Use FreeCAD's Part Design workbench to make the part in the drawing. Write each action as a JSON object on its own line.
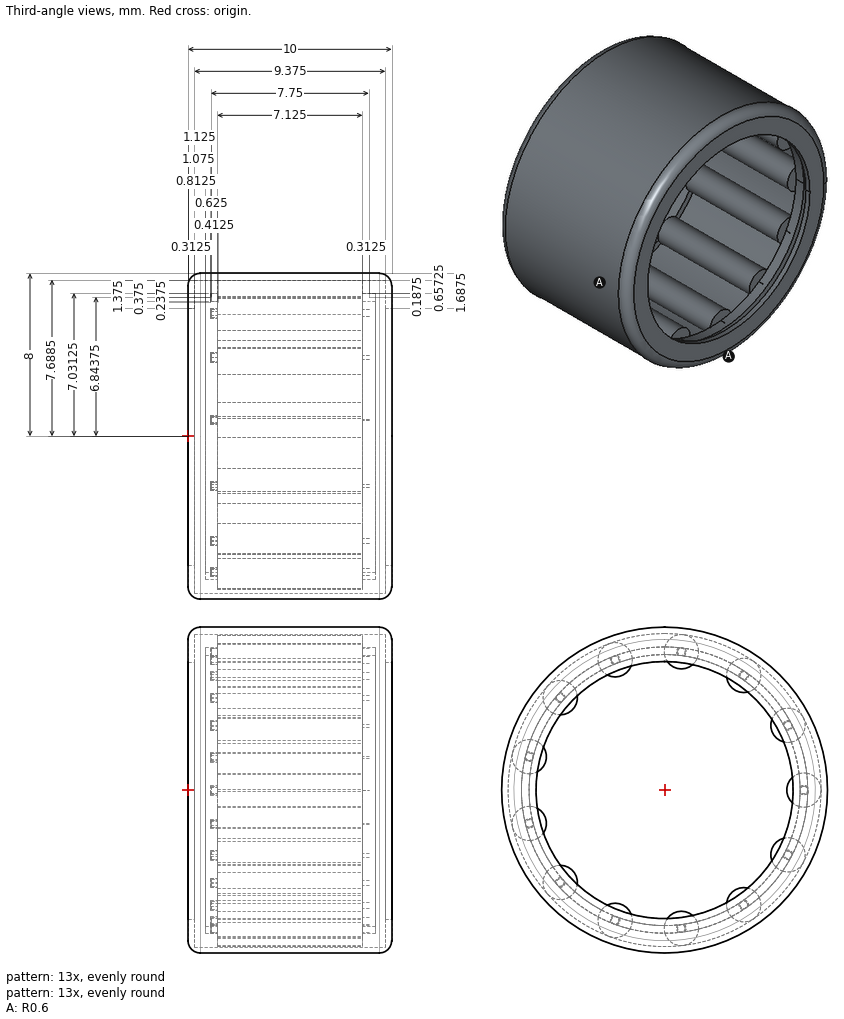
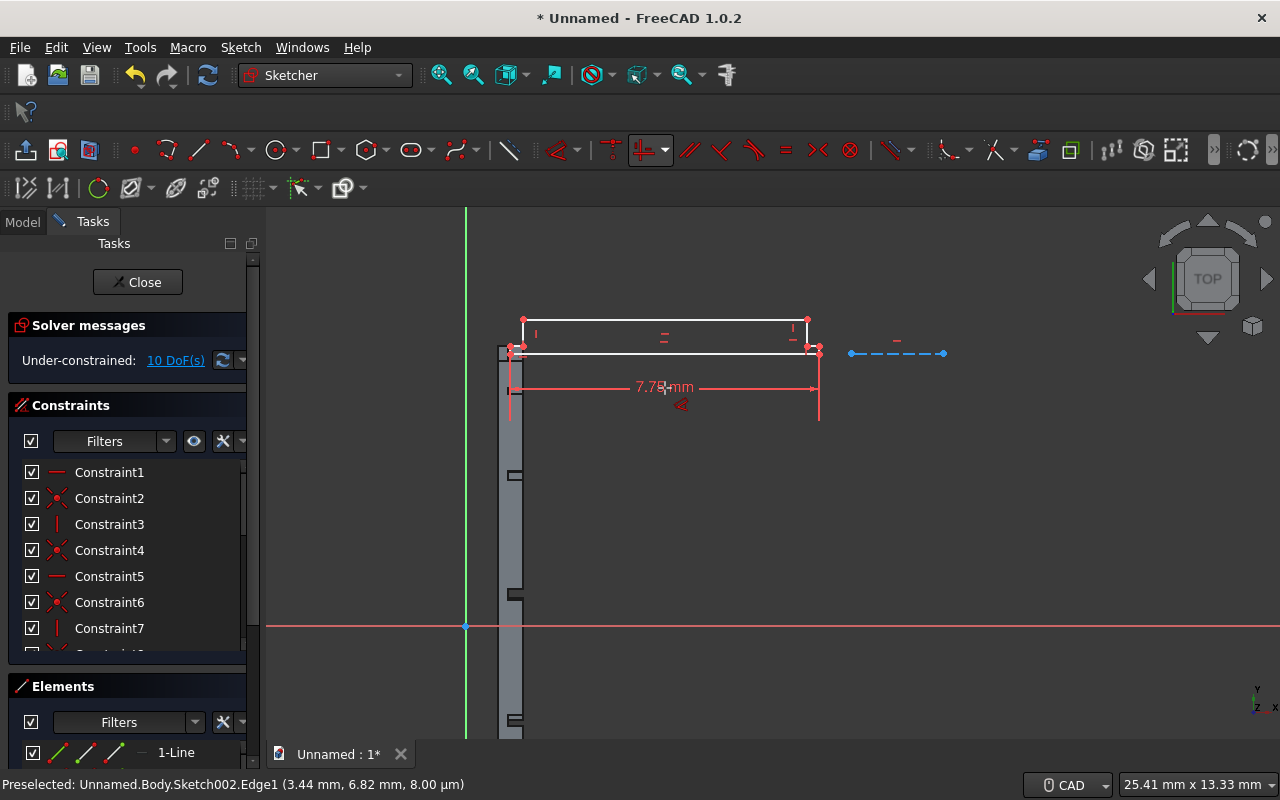
{"action": "left_click", "coordinate": [722, 320]}
{"action": "left_click", "coordinate": [665, 286]}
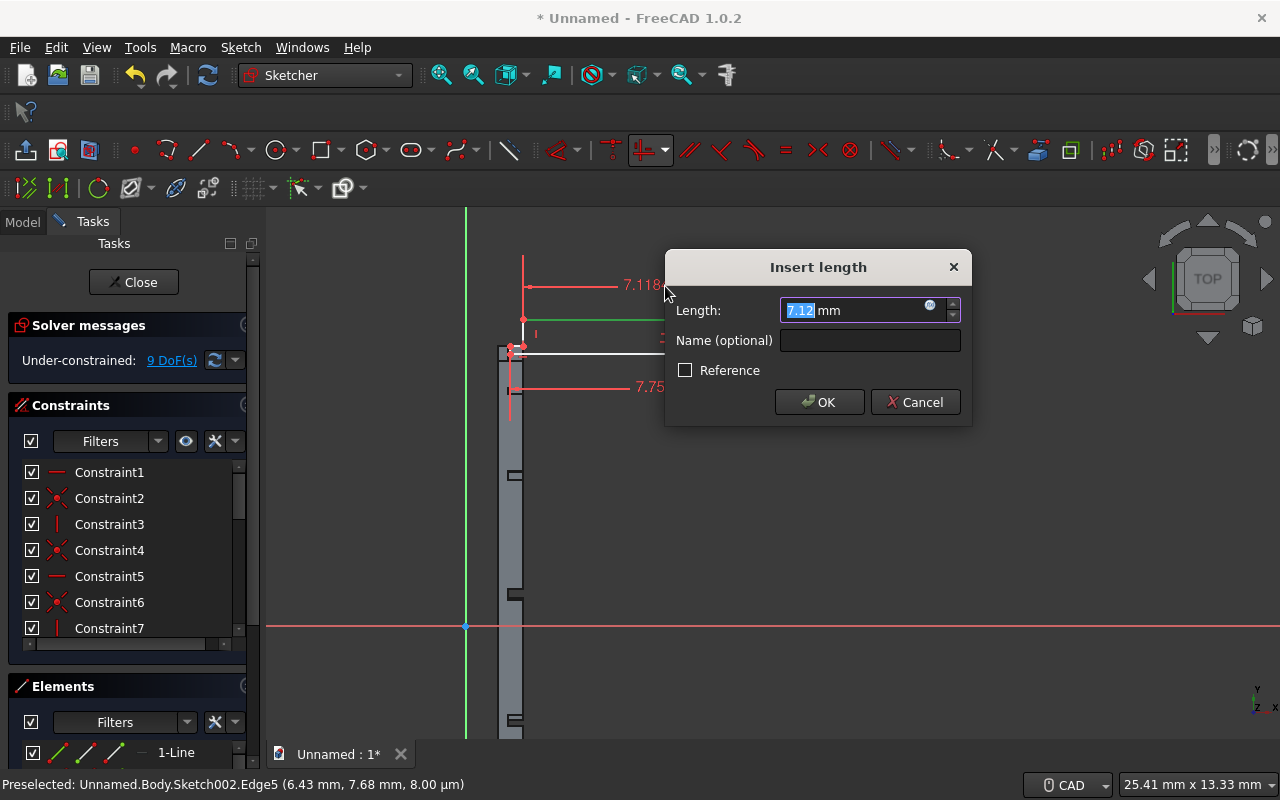
{"action": "type", "text": "7.125"}
{"action": "key", "text": "Return"}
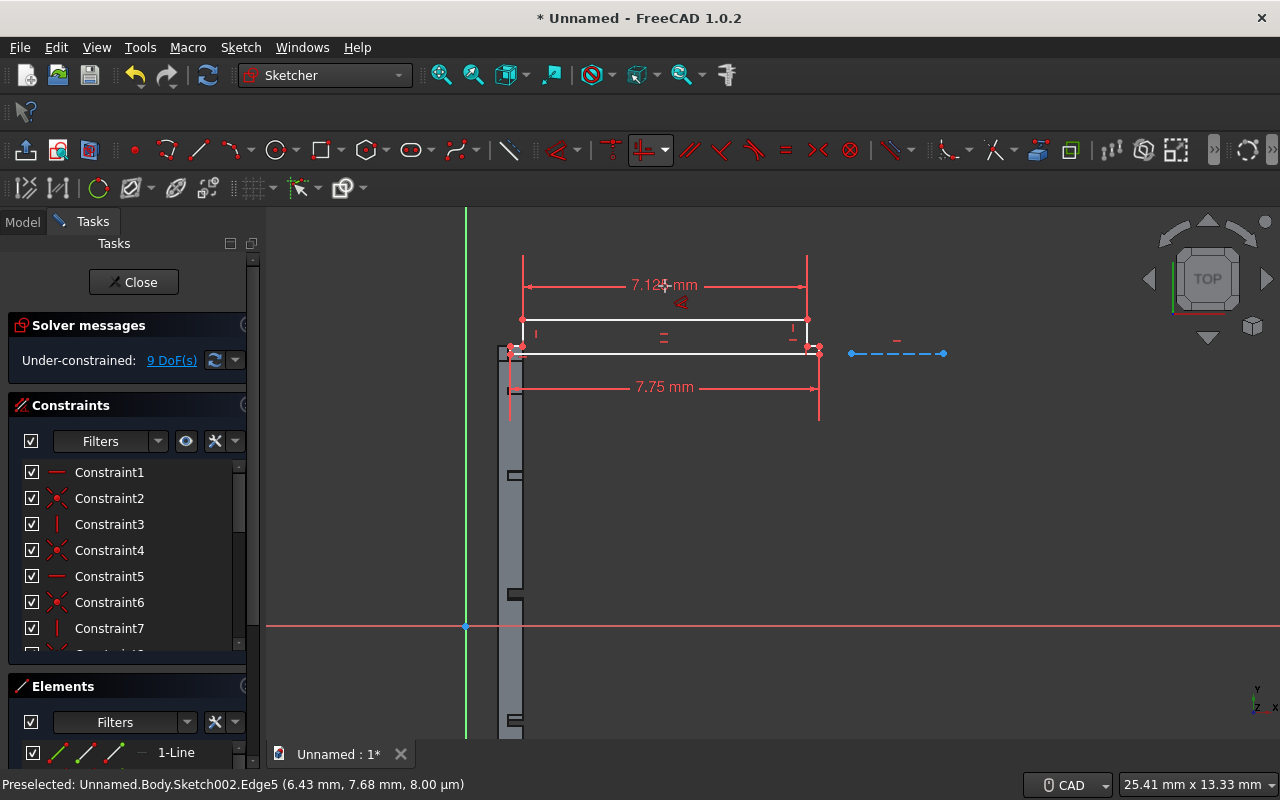
{"action": "scroll", "coordinate": [819, 350], "scroll_direction": "up", "scroll_amount": 9}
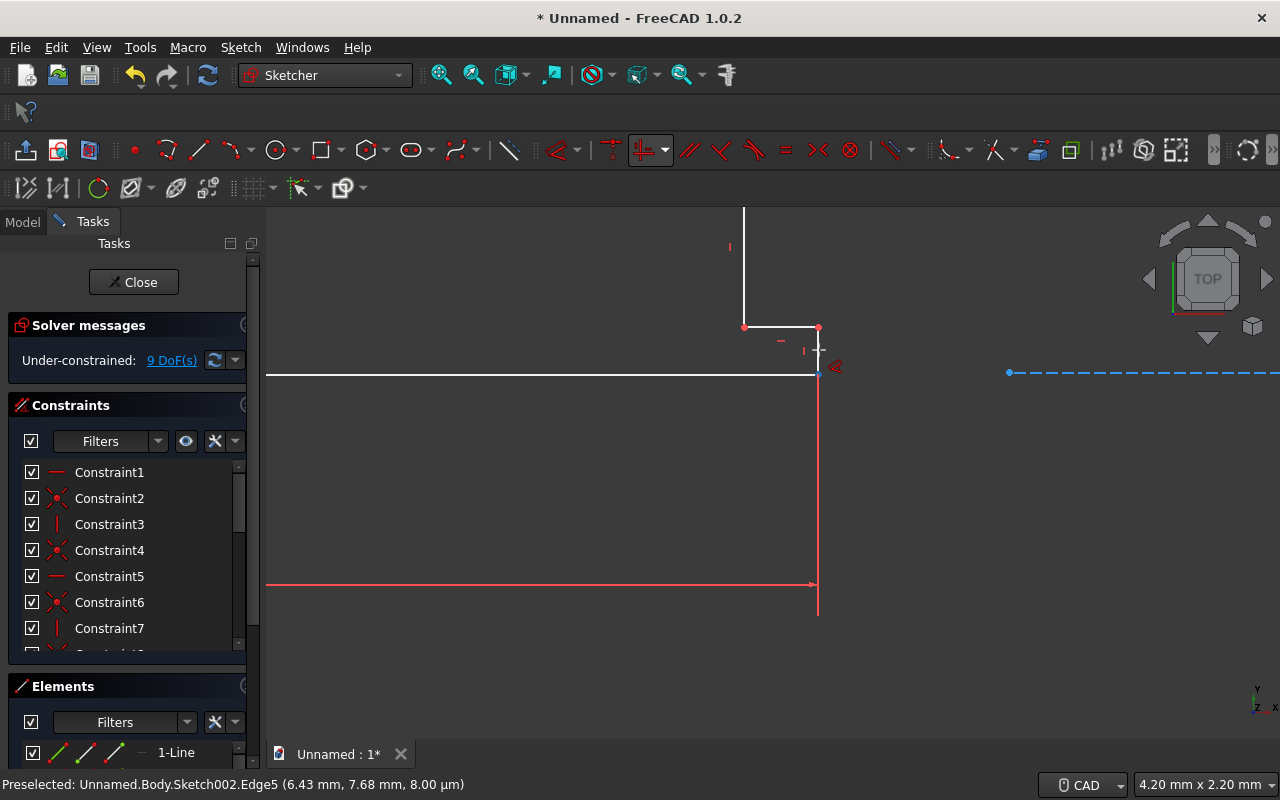
{"action": "left_click", "coordinate": [818, 351]}
{"action": "left_click", "coordinate": [852, 351]}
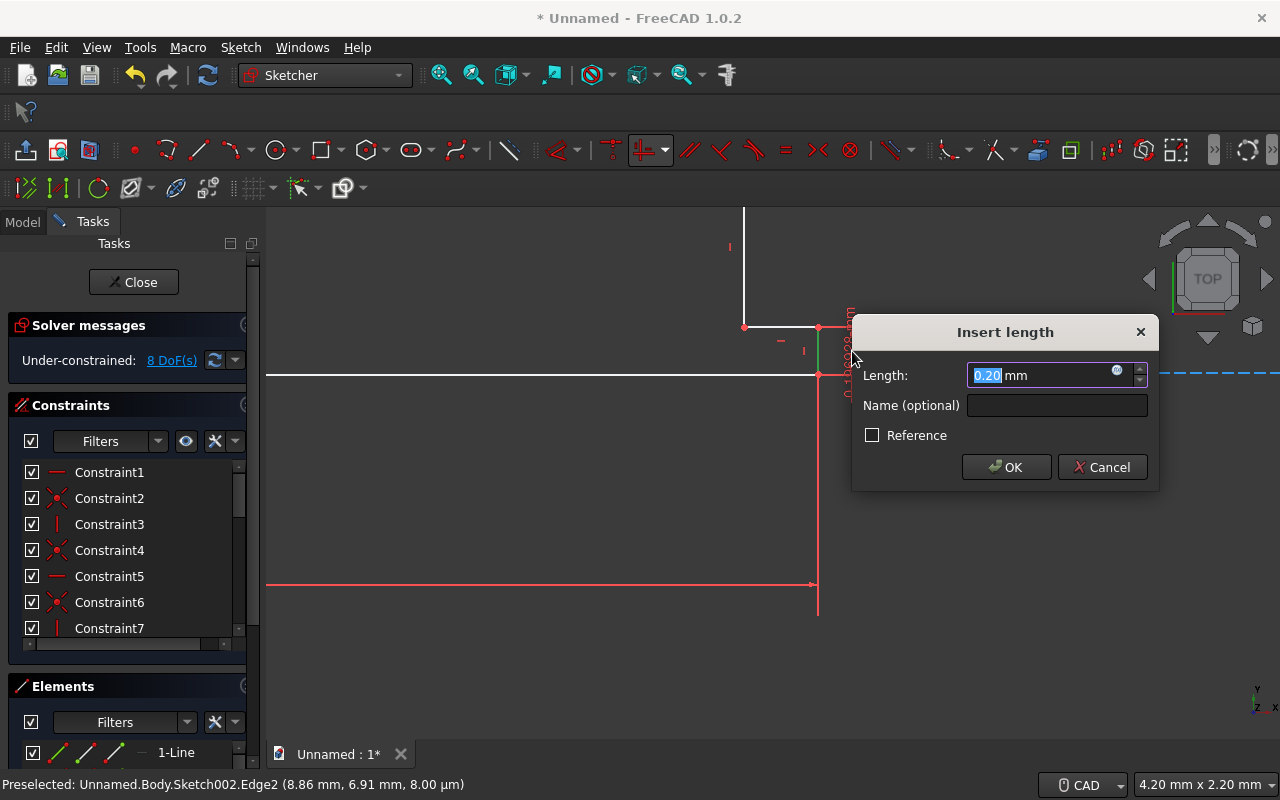
{"action": "type", "text": "0.1875"}
{"action": "key", "text": "Return"}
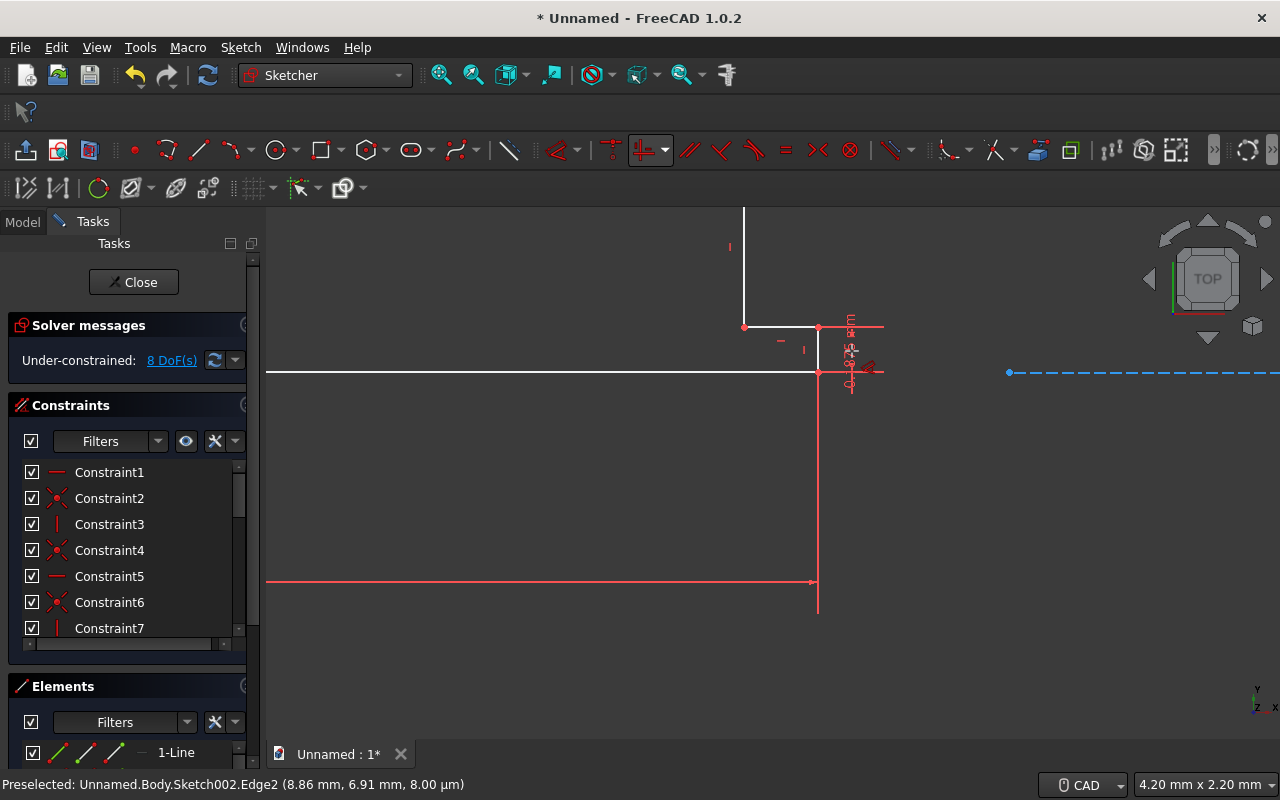
{"action": "left_click", "coordinate": [796, 327]}
{"action": "left_click", "coordinate": [781, 293]}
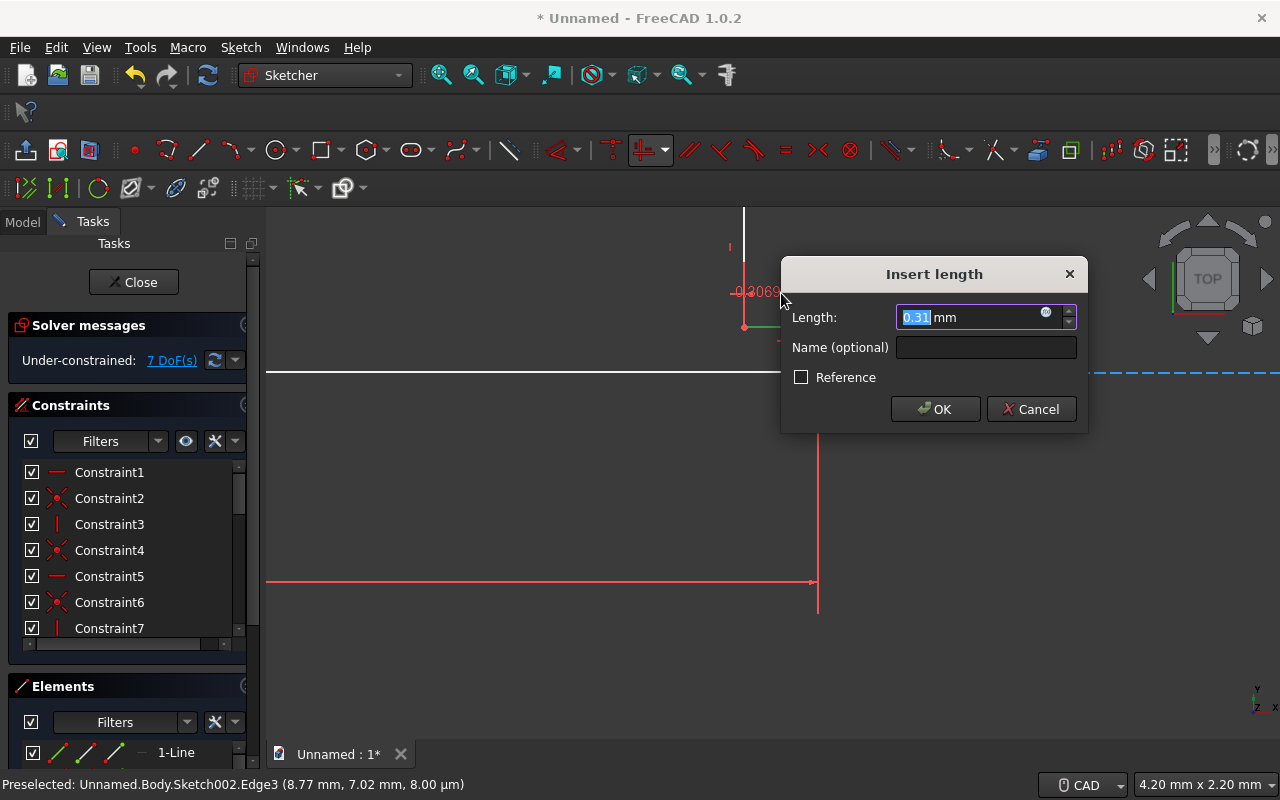
{"action": "type", "text": "0.3125"}
{"action": "key", "text": "Return"}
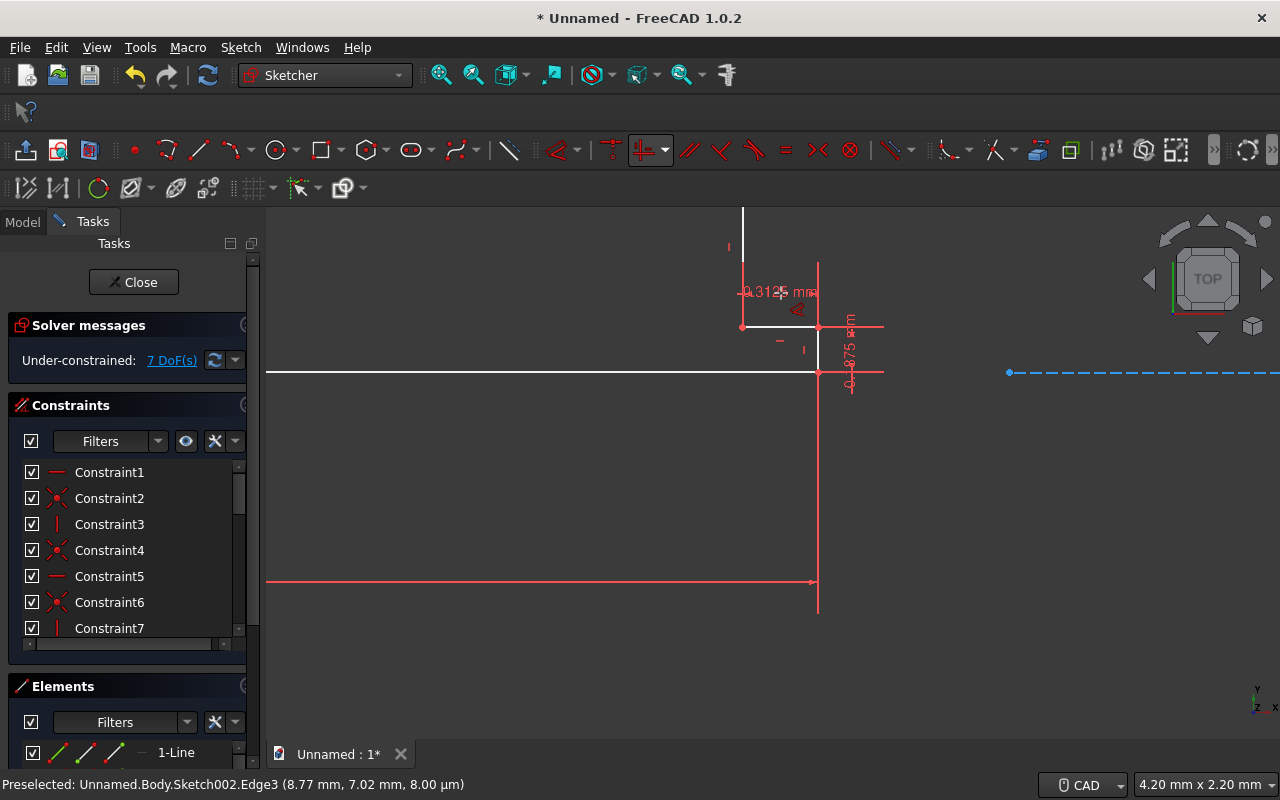
{"action": "scroll", "coordinate": [820, 350], "scroll_direction": "down", "scroll_amount": 9}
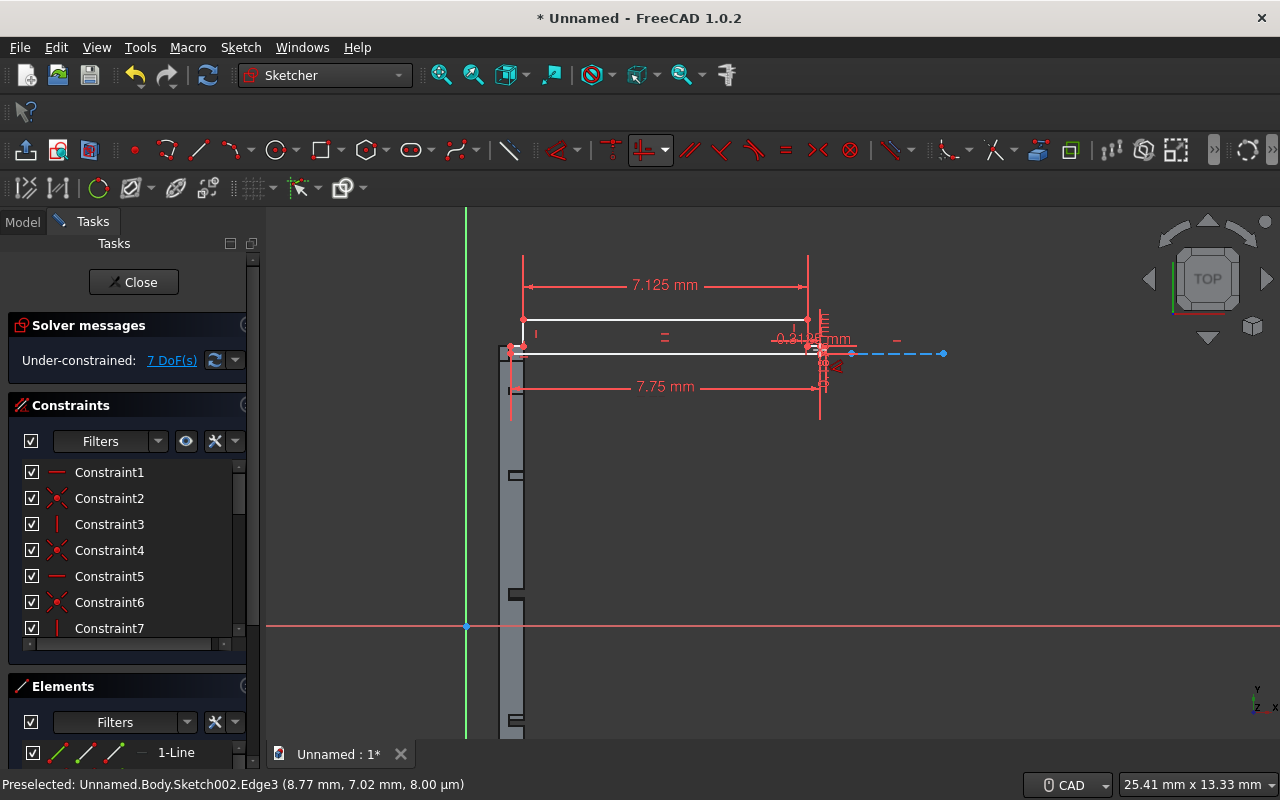
{"action": "scroll", "coordinate": [511, 348], "scroll_direction": "up", "scroll_amount": 9}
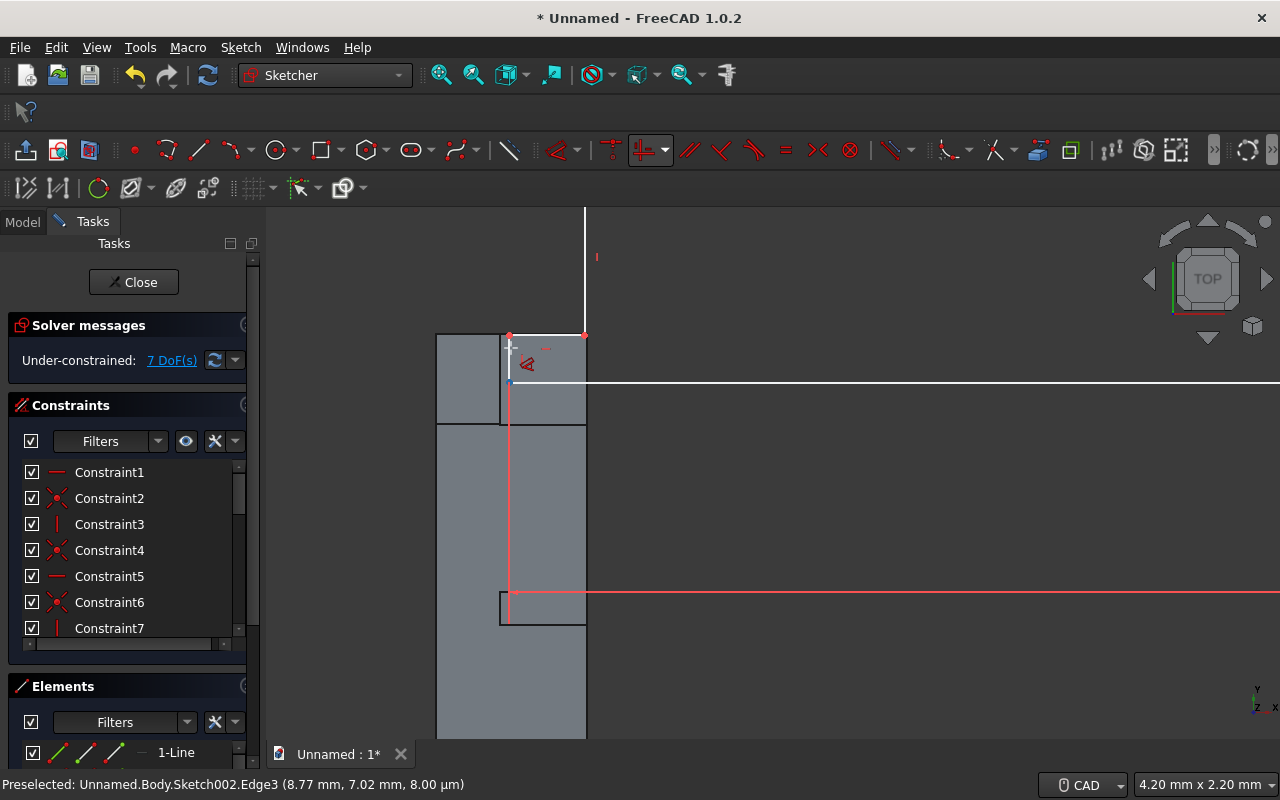
{"action": "left_click", "coordinate": [509, 350]}
{"action": "left_click", "coordinate": [475, 359]}